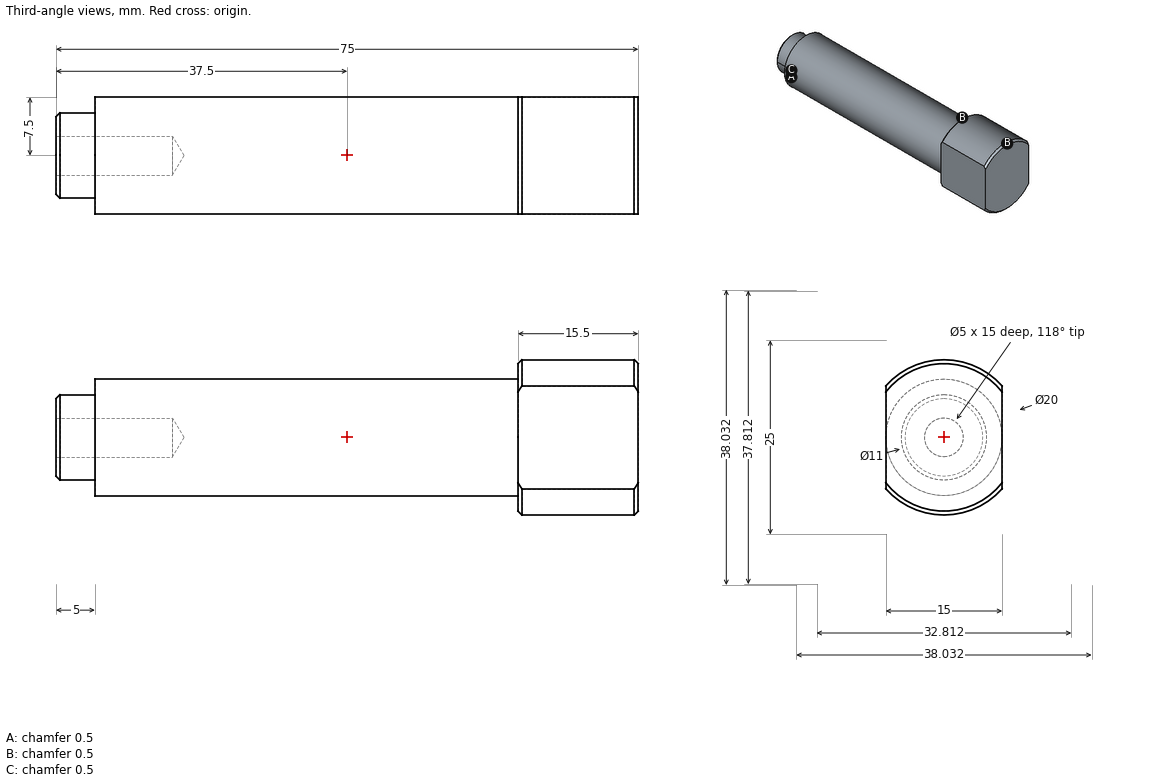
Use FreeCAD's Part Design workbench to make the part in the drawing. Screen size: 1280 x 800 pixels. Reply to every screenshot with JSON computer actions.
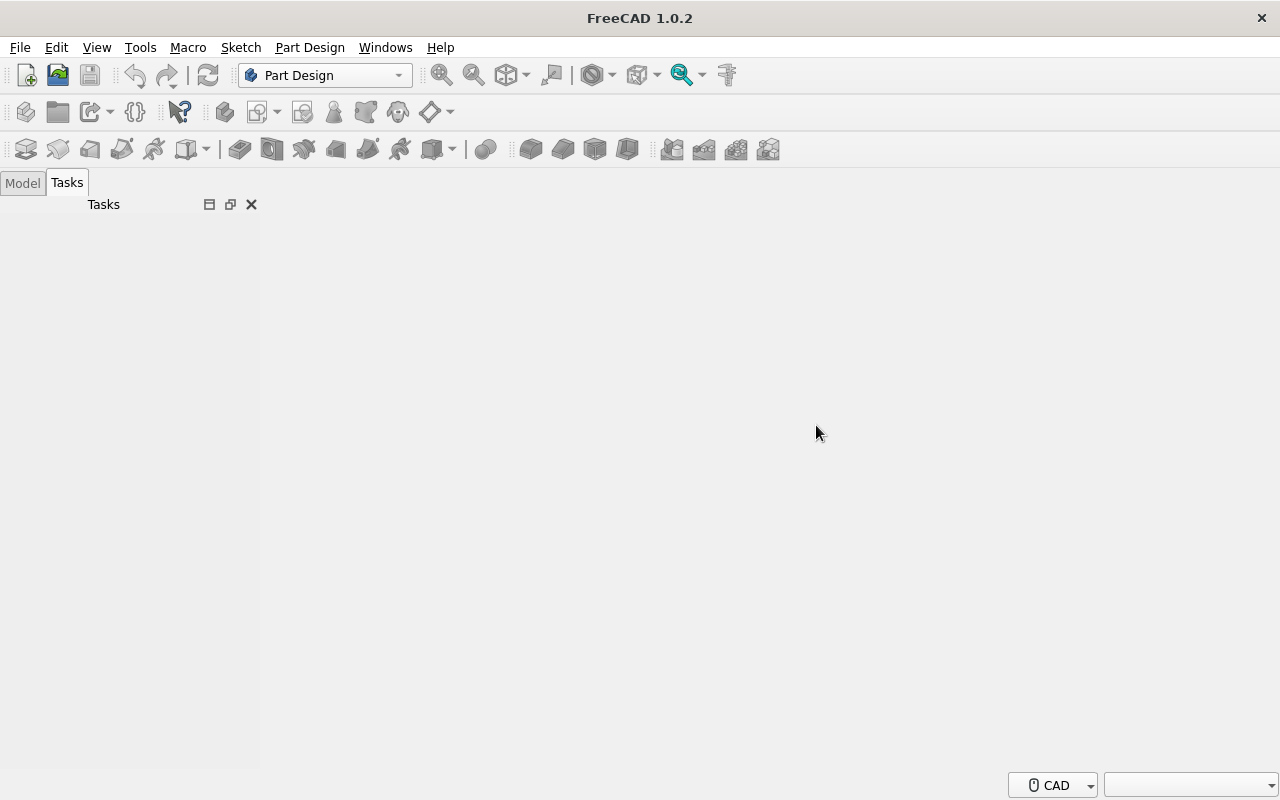
{"action": "left_click", "coordinate": [26, 76]}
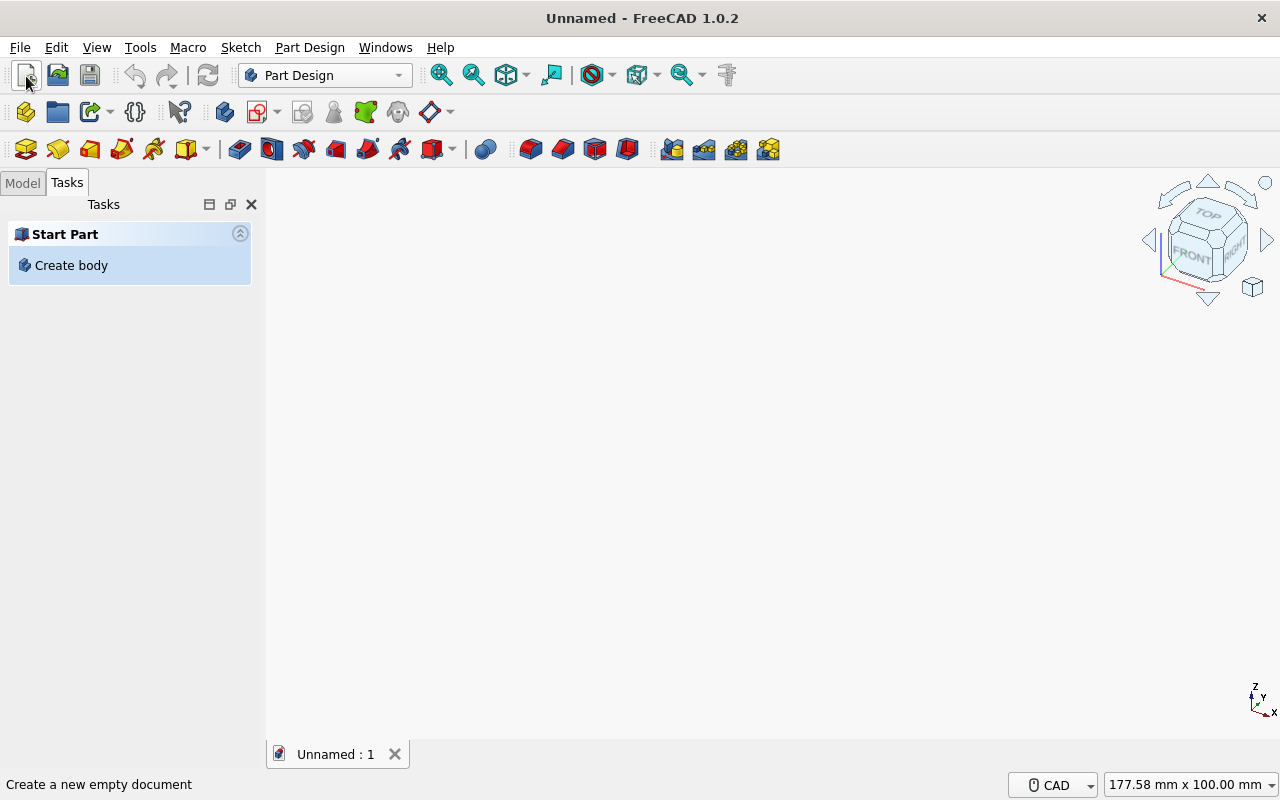
{"action": "left_click", "coordinate": [258, 112]}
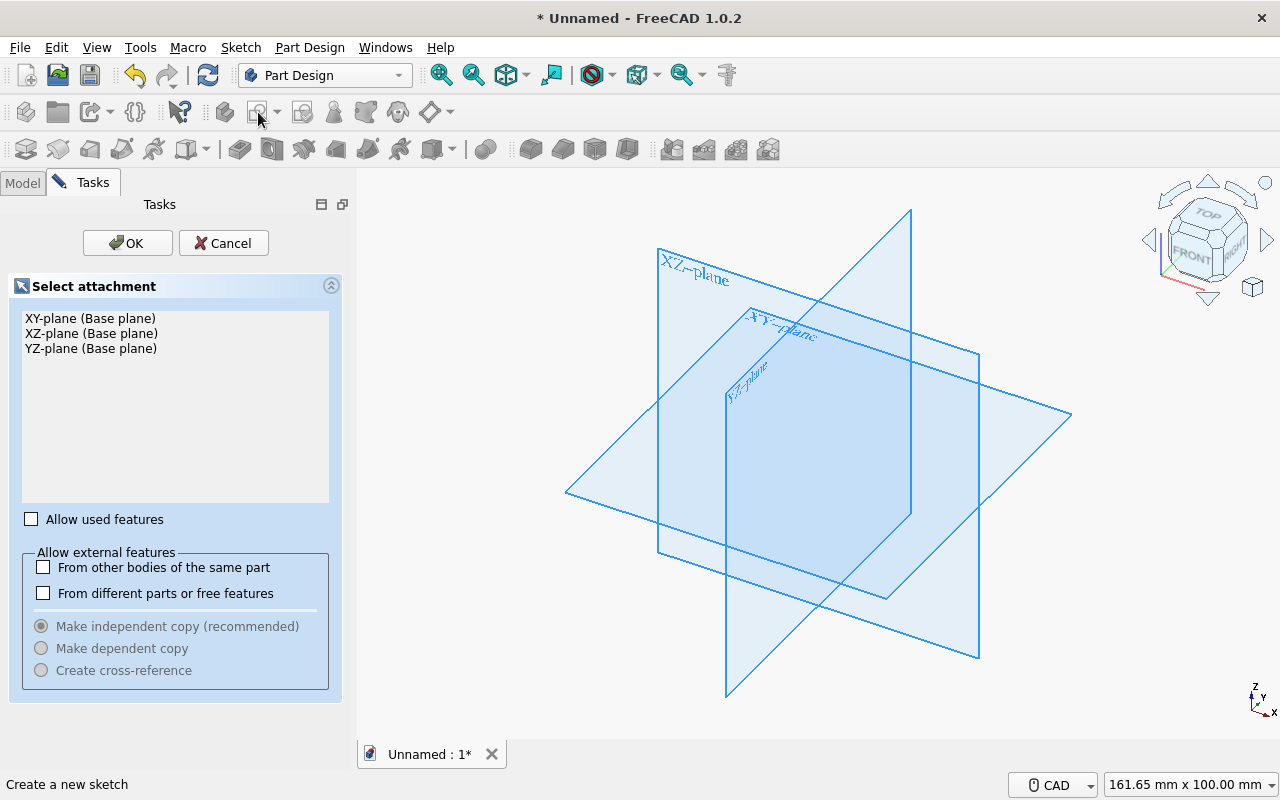
{"action": "left_click", "coordinate": [82, 318]}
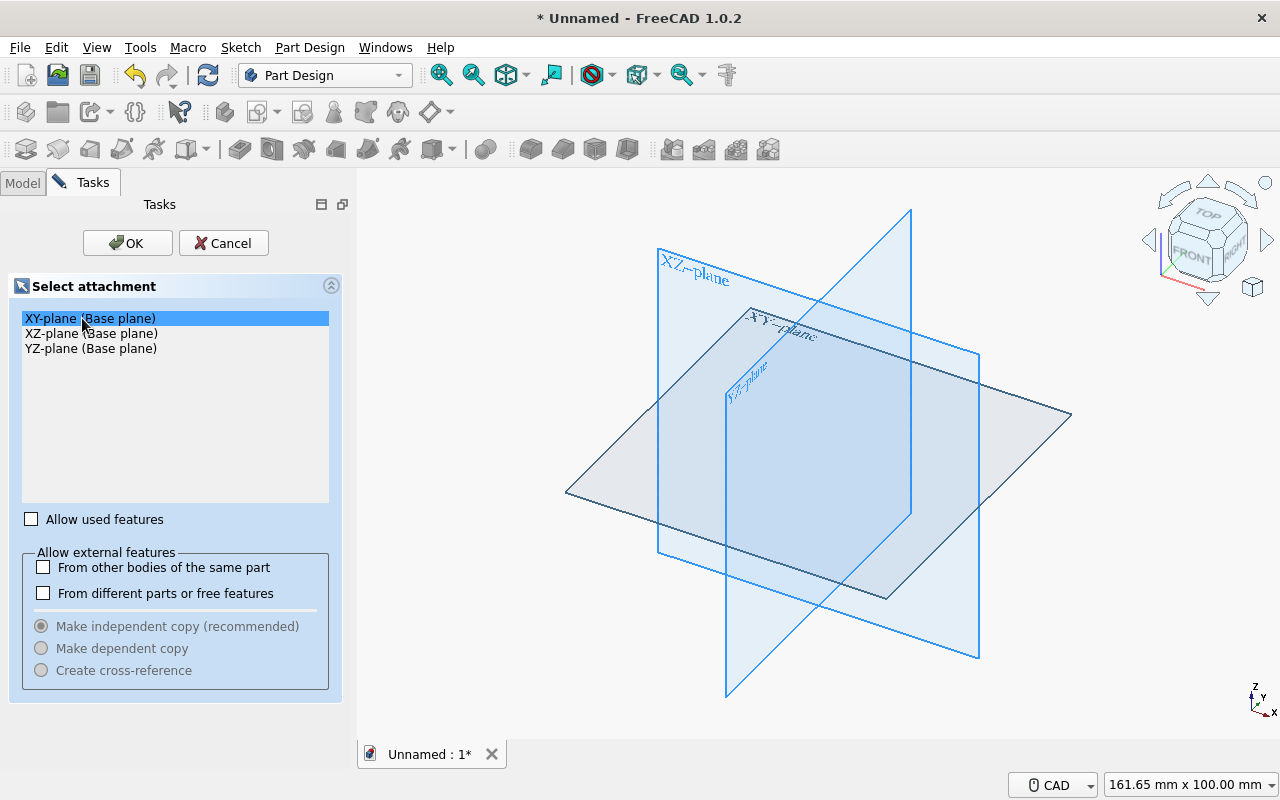
{"action": "left_click", "coordinate": [128, 243]}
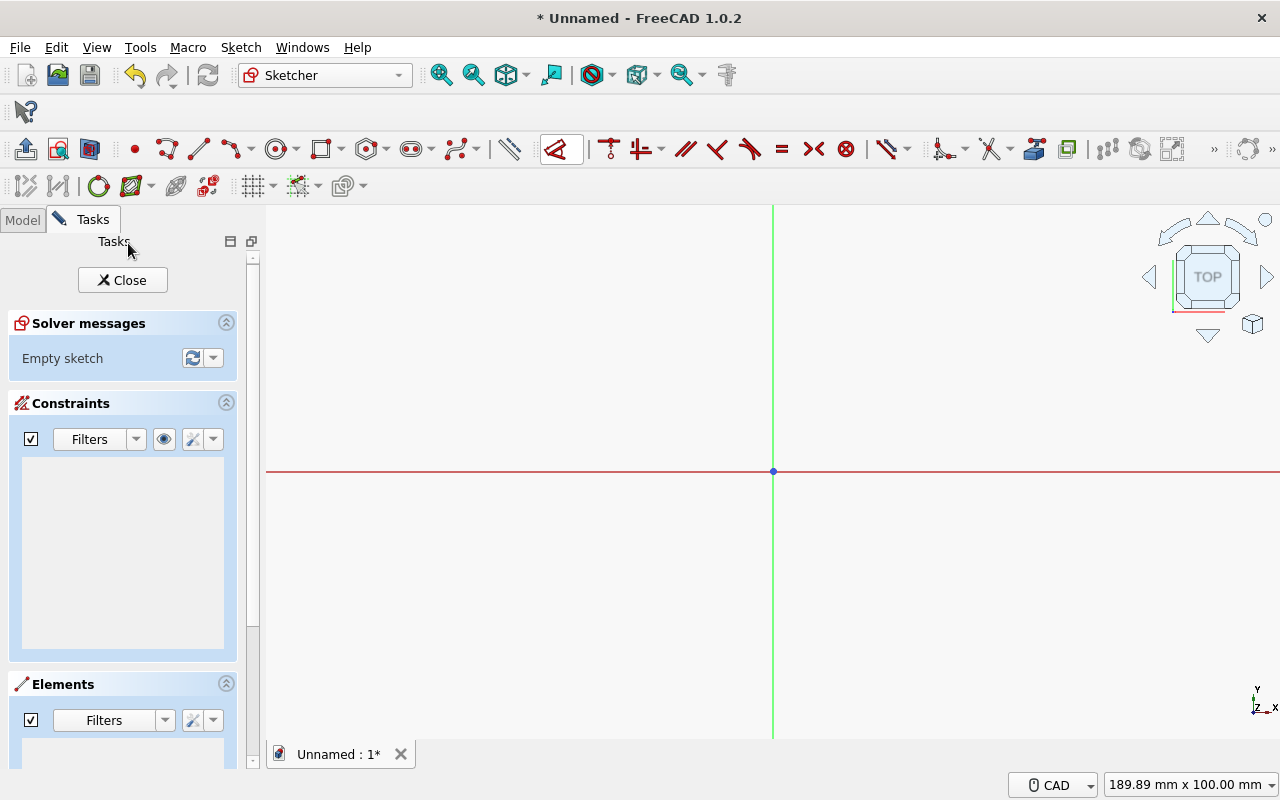
{"action": "scroll", "coordinate": [912, 411], "scroll_direction": "up", "scroll_amount": 2}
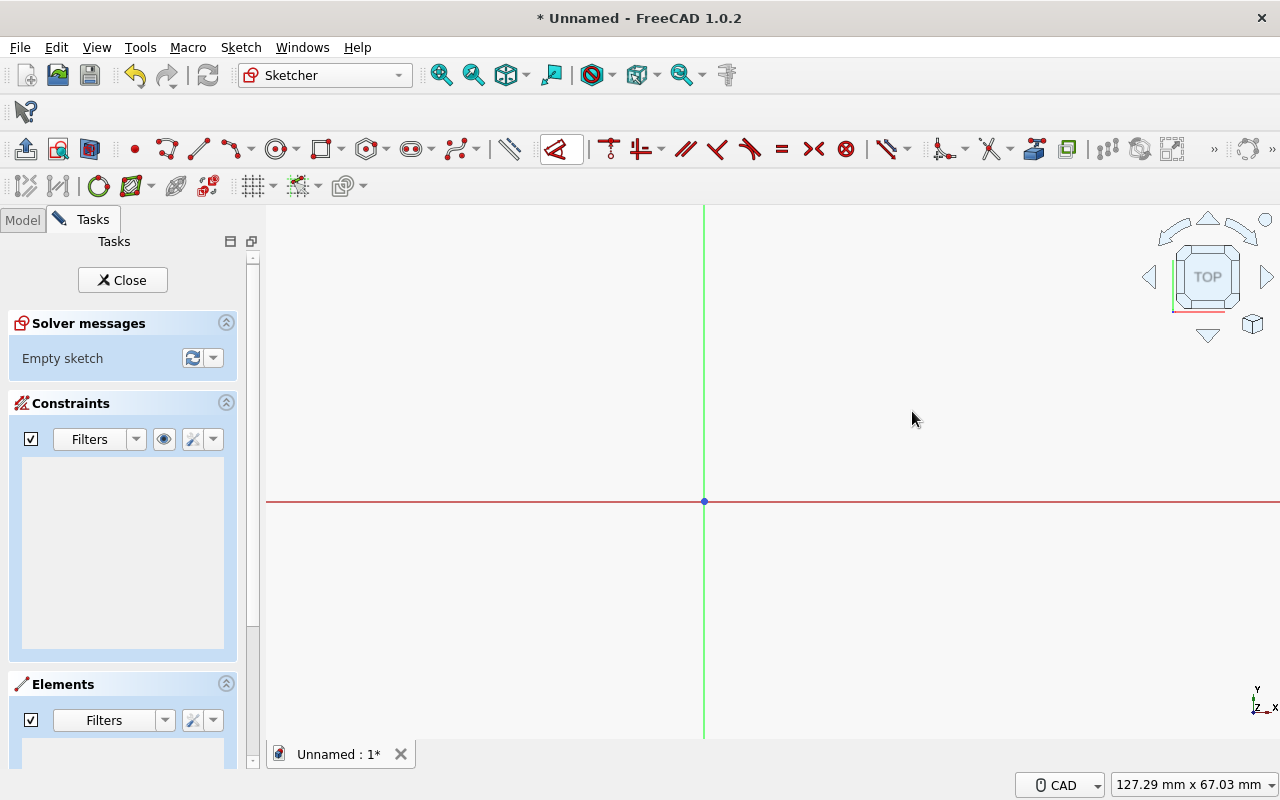
{"action": "left_click", "coordinate": [322, 150]}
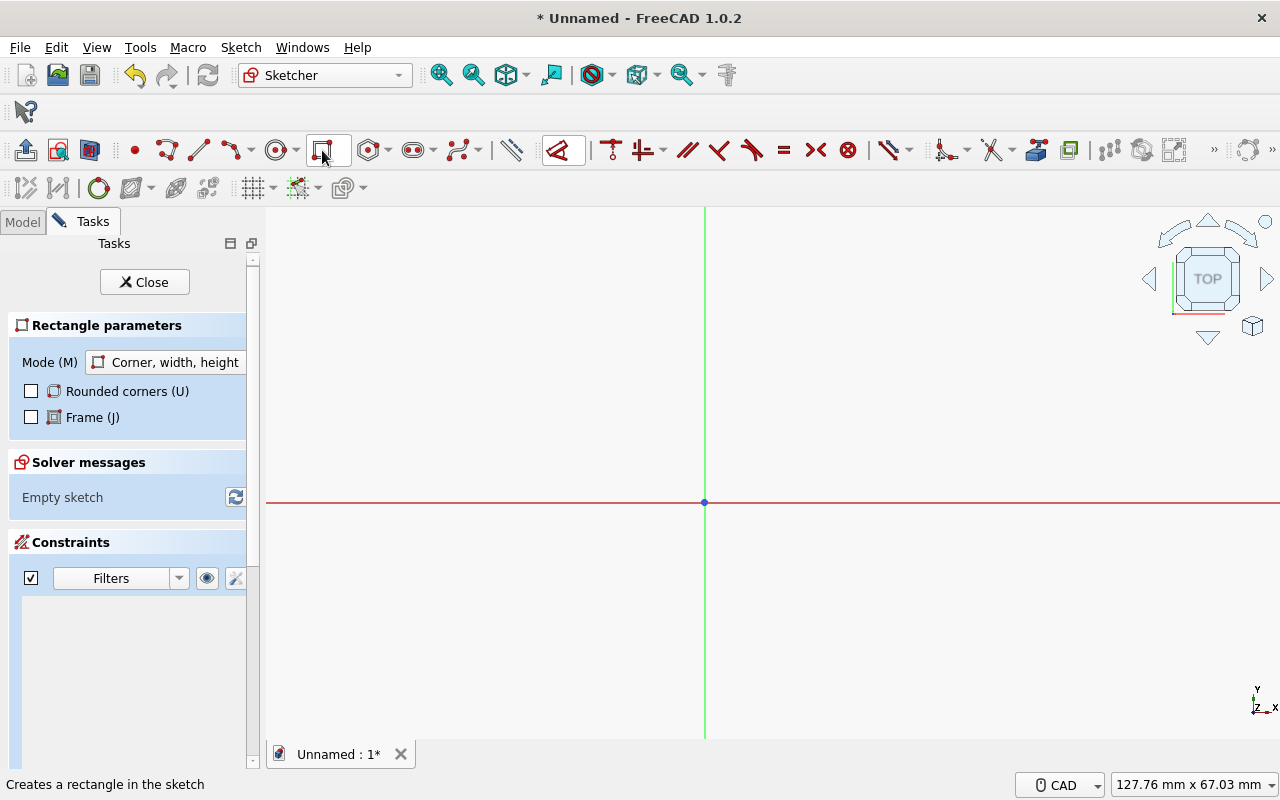
{"action": "left_click", "coordinate": [407, 443]}
{"action": "left_click", "coordinate": [1002, 503]}
{"action": "key", "text": "Escape"}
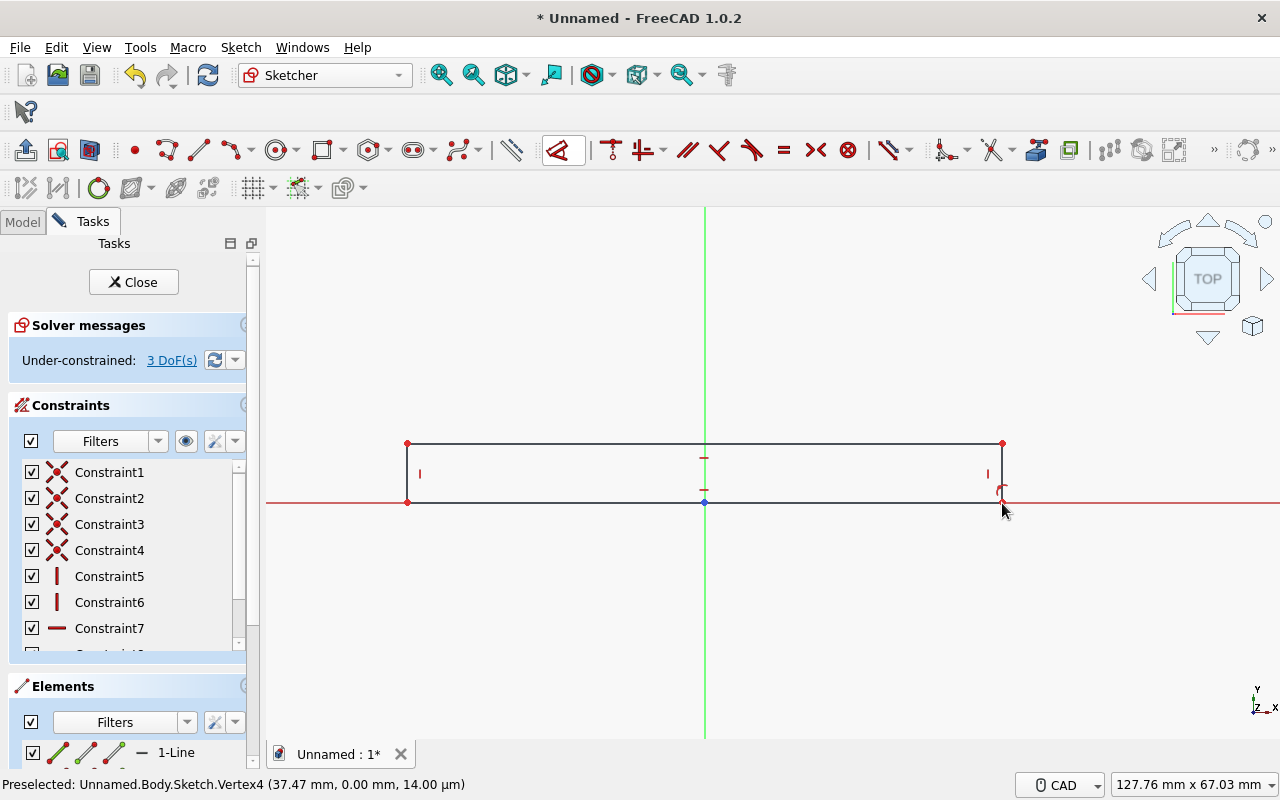
{"action": "left_click", "coordinate": [558, 150]}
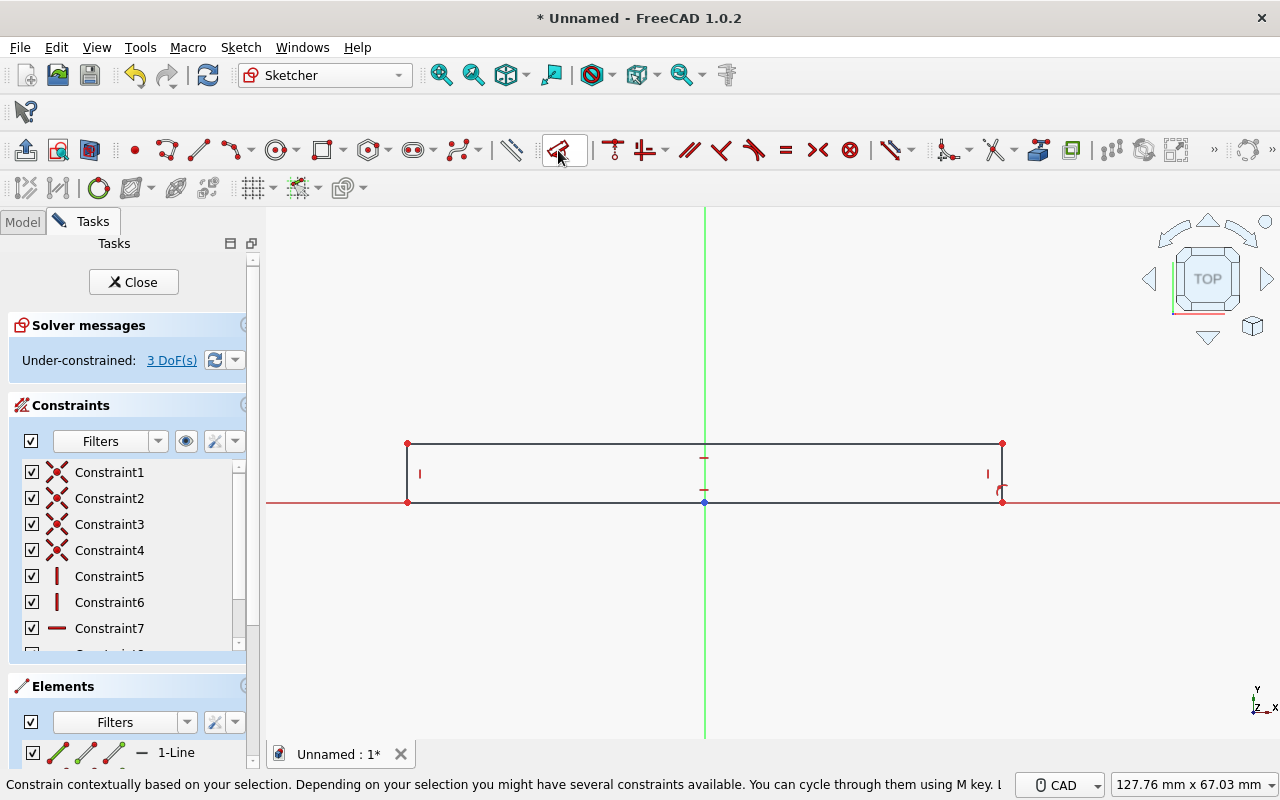
{"action": "left_click", "coordinate": [585, 503]}
{"action": "left_click", "coordinate": [568, 537]}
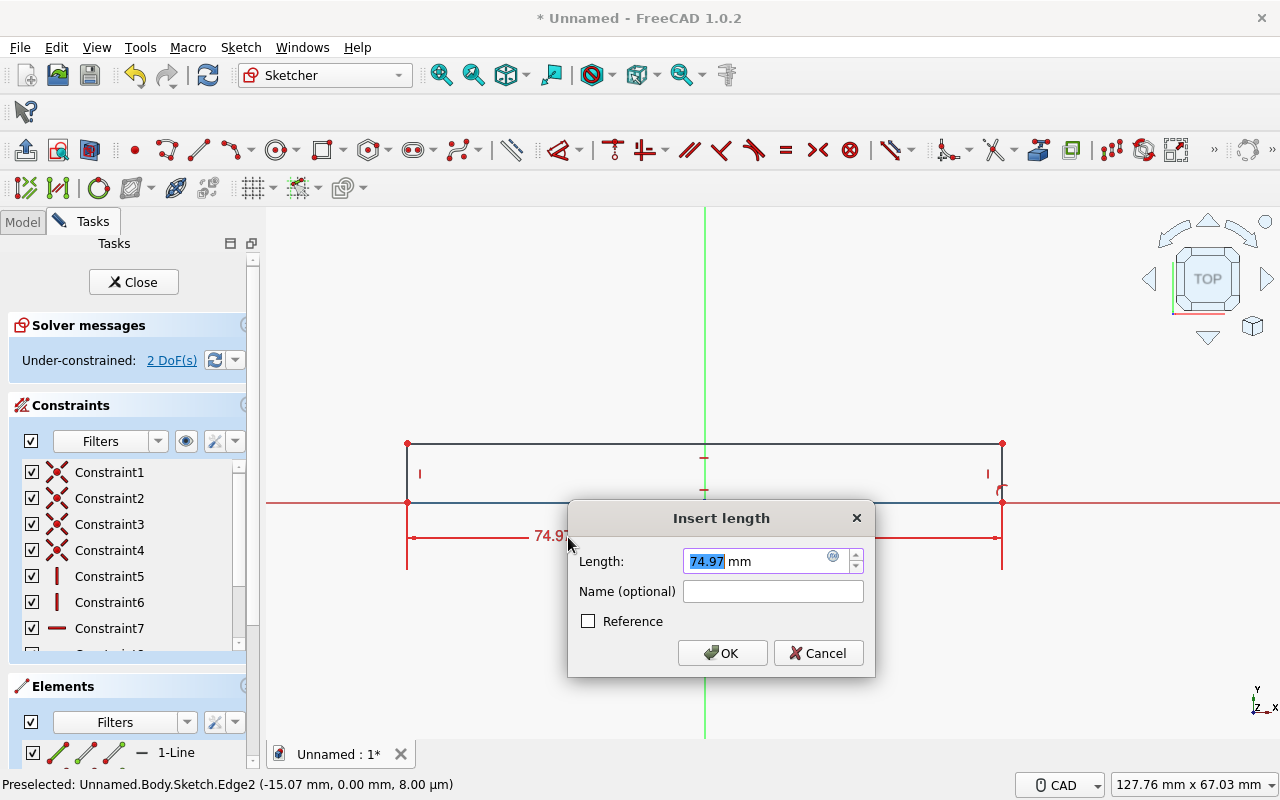
{"action": "type", "text": "75"}
{"action": "key", "text": "Return"}